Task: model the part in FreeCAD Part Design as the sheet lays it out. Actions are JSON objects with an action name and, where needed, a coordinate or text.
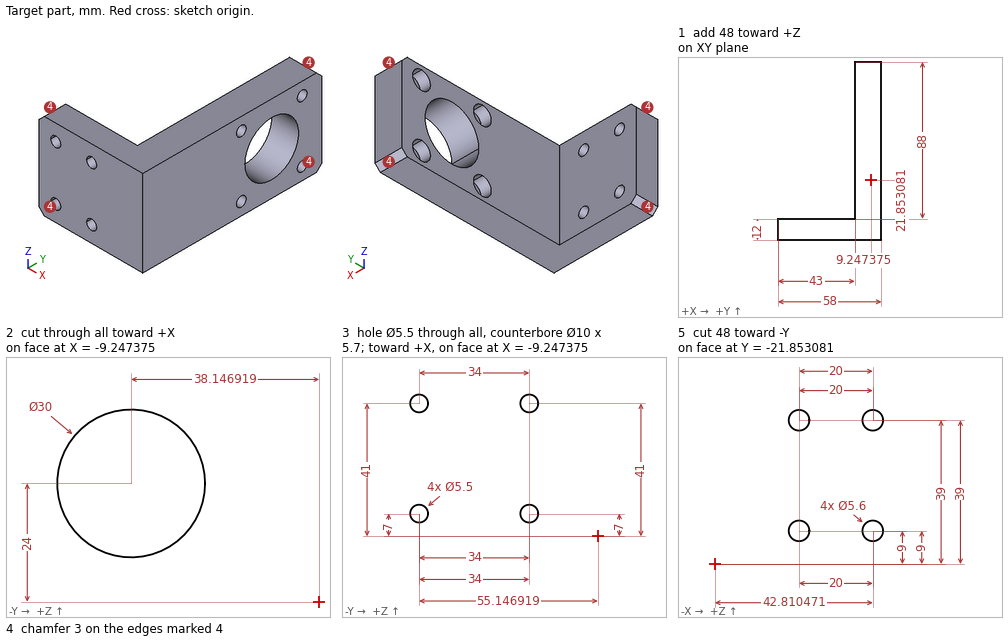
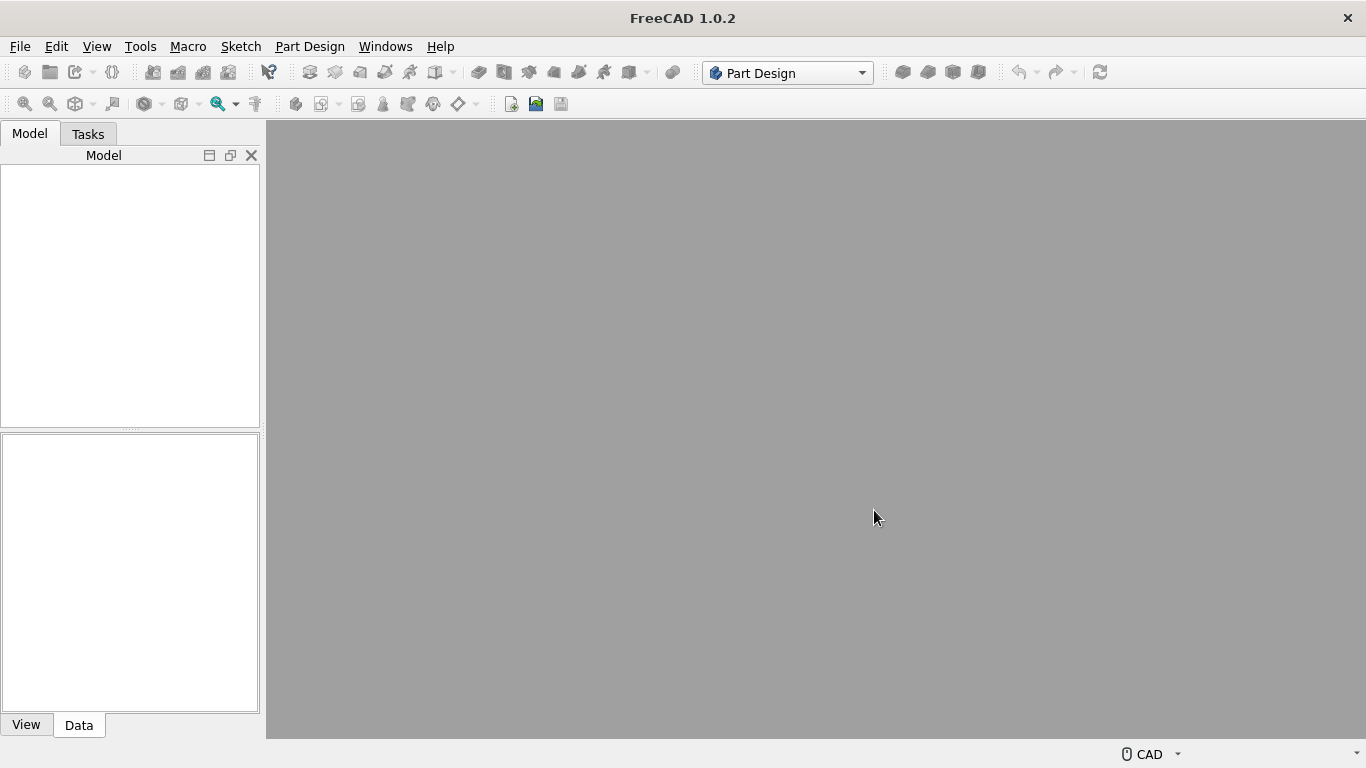
{"action": "left_click", "coordinate": [511, 104]}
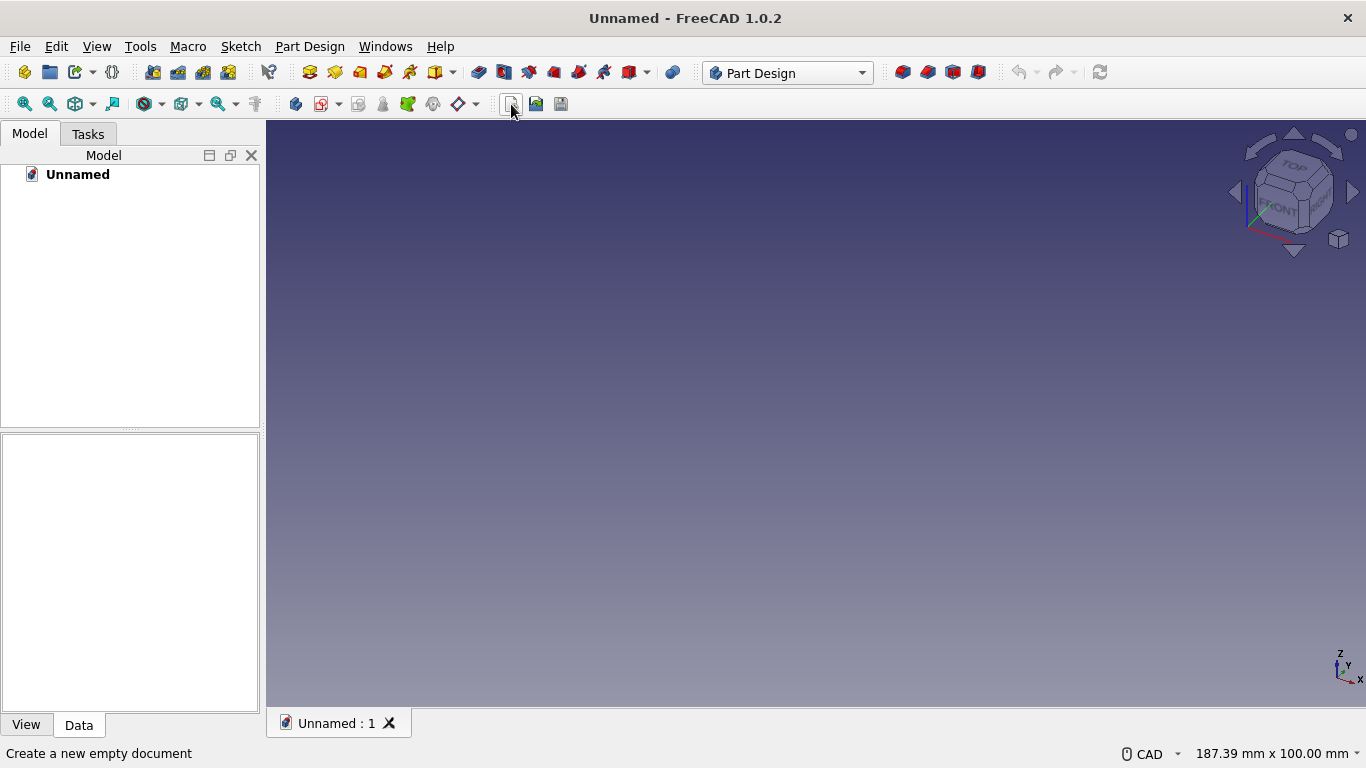
{"action": "left_click", "coordinate": [320, 104]}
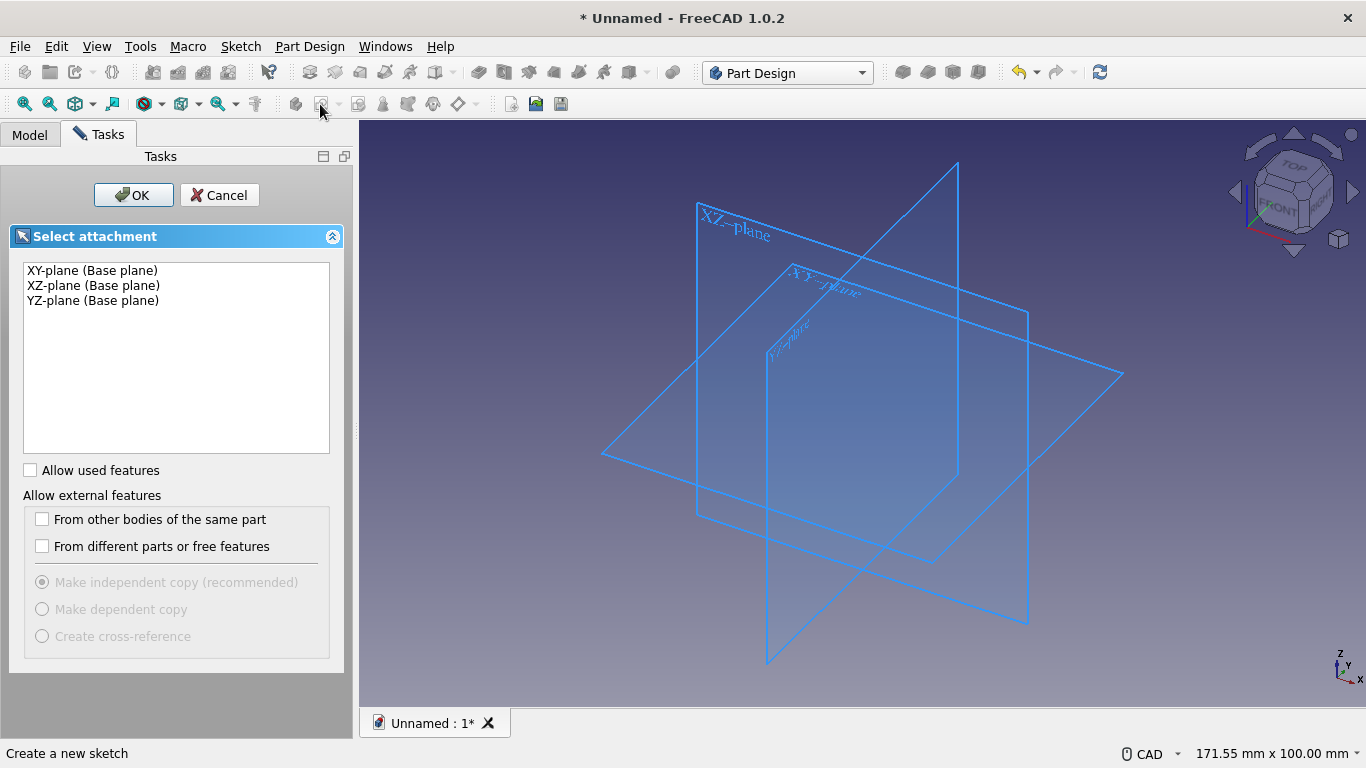
{"action": "left_click", "coordinate": [84, 270]}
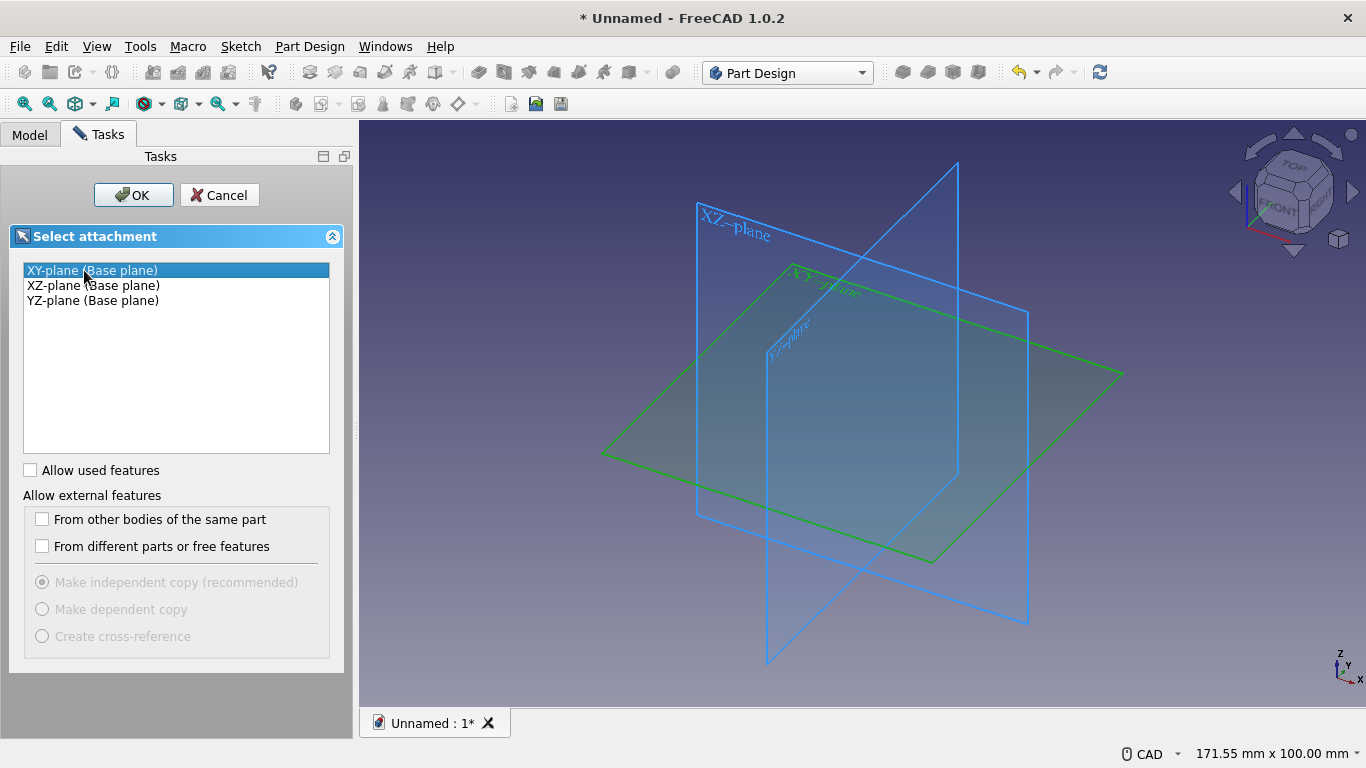
{"action": "left_click", "coordinate": [134, 195]}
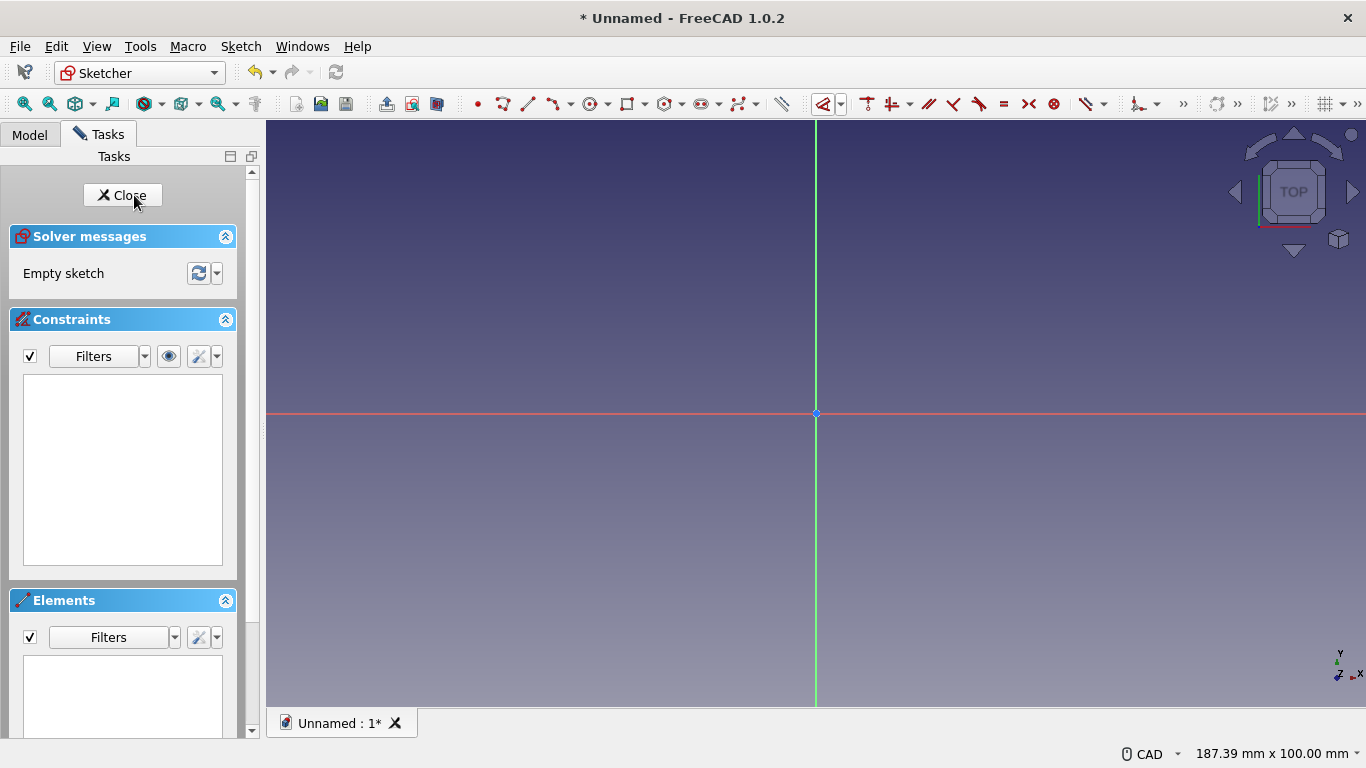
{"action": "scroll", "coordinate": [886, 606], "scroll_direction": "down", "scroll_amount": 2}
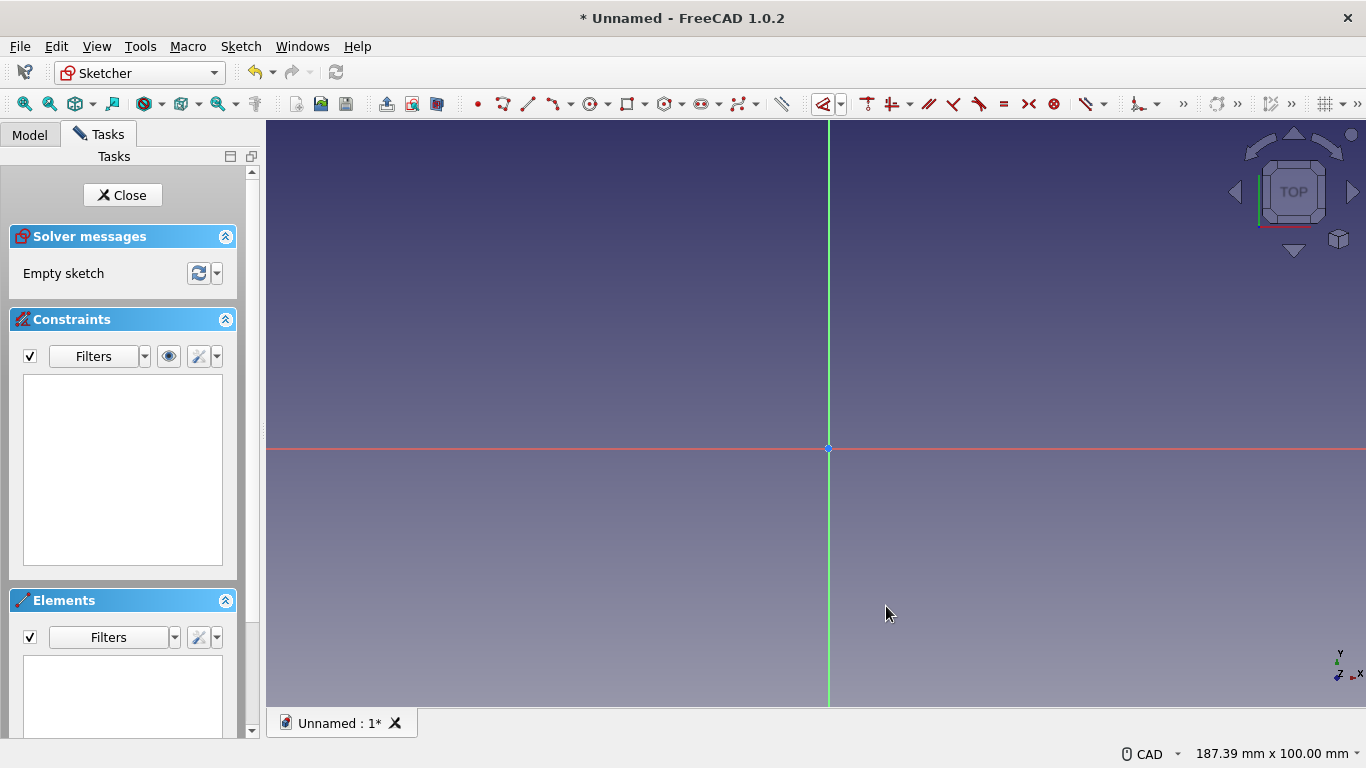
{"action": "left_click", "coordinate": [503, 104]}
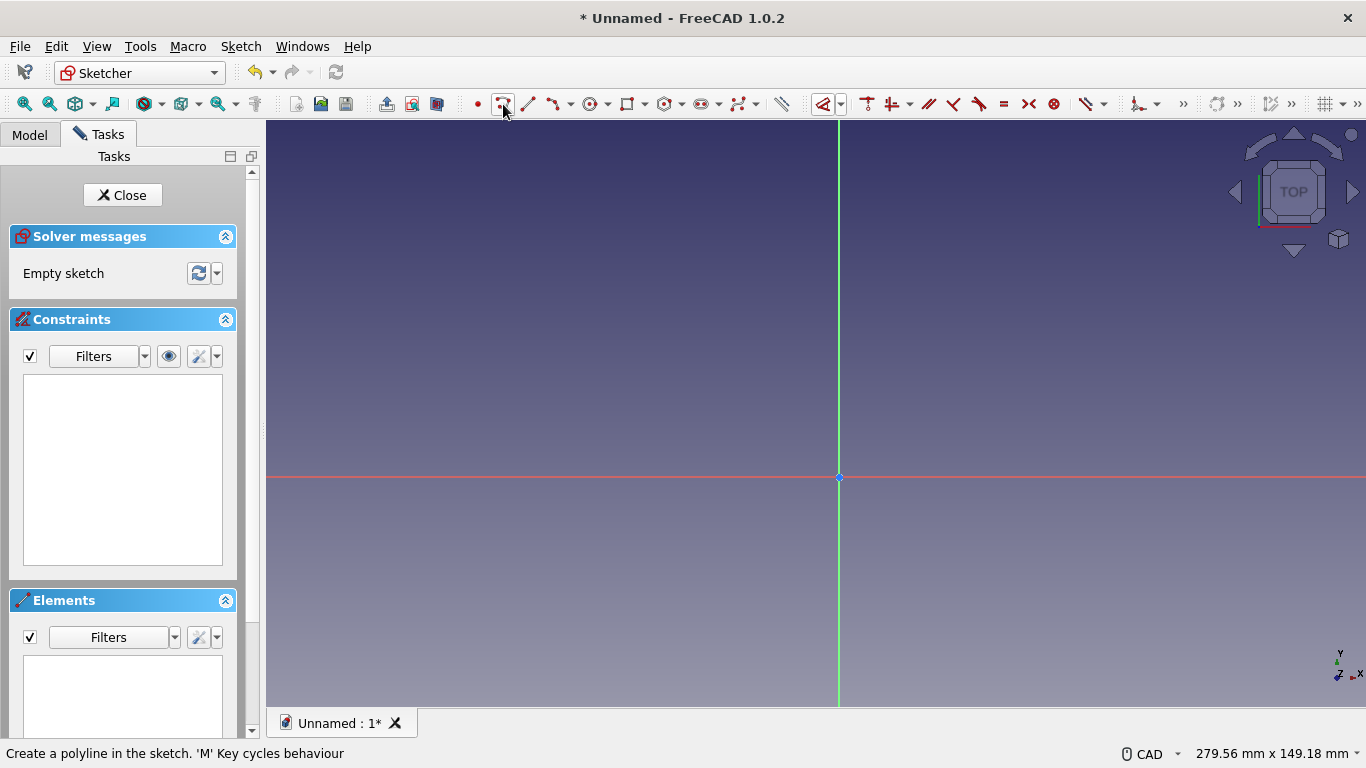
{"action": "left_click", "coordinate": [803, 563]}
{"action": "left_click", "coordinate": [634, 563]}
{"action": "left_click", "coordinate": [634, 610]}
{"action": "left_click", "coordinate": [862, 610]}
{"action": "left_click", "coordinate": [862, 217]}
{"action": "left_click", "coordinate": [803, 217]}
{"action": "left_click", "coordinate": [803, 564]}
{"action": "key", "text": "Escape"}
{"action": "key", "text": "Escape"}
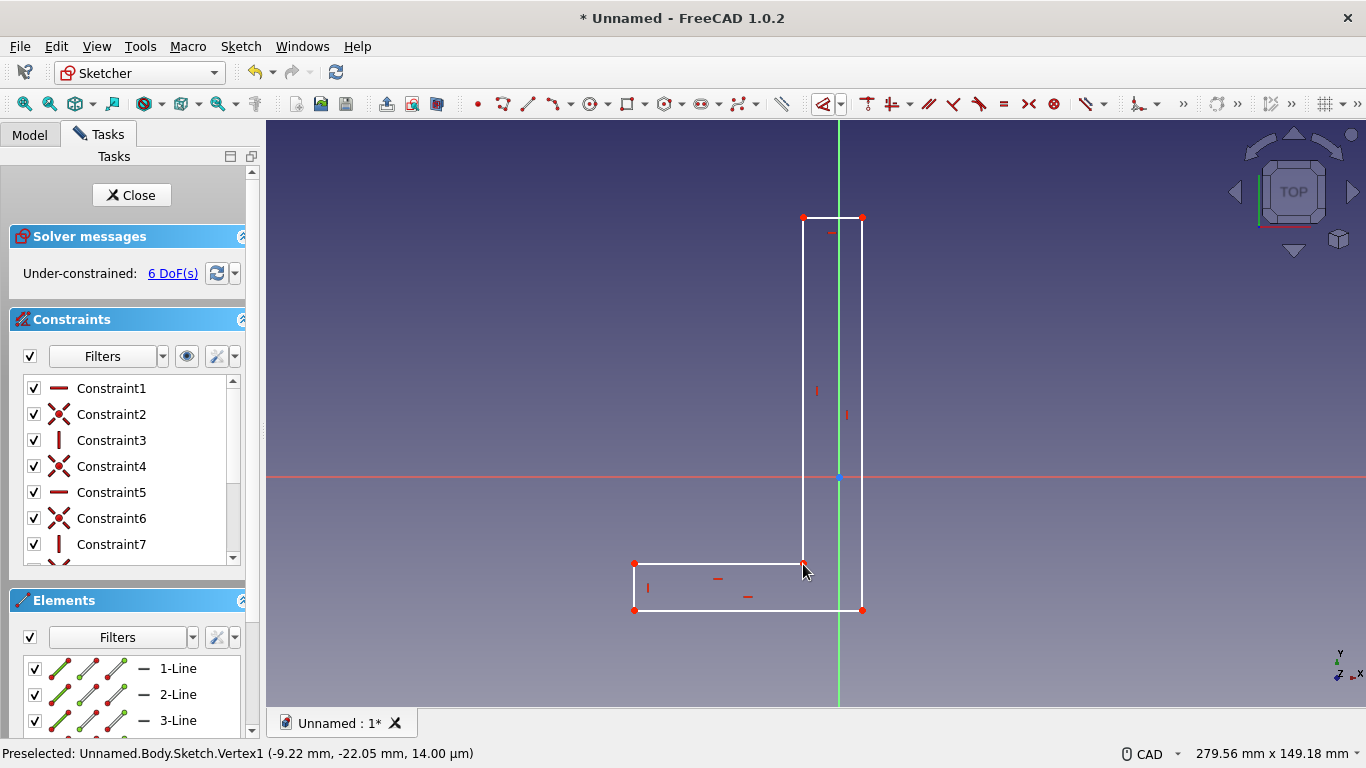
{"action": "left_click", "coordinate": [822, 104]}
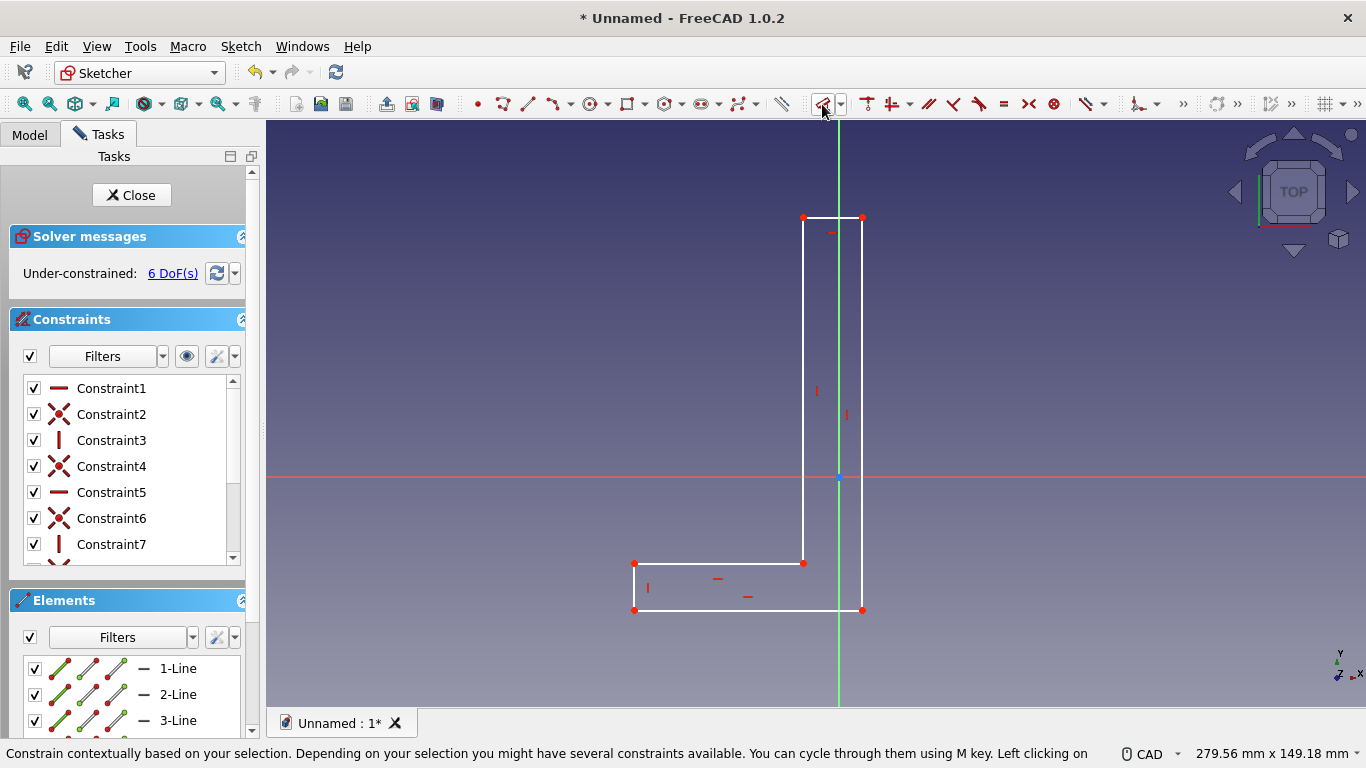
{"action": "left_click", "coordinate": [752, 564]}
{"action": "left_click", "coordinate": [719, 530]}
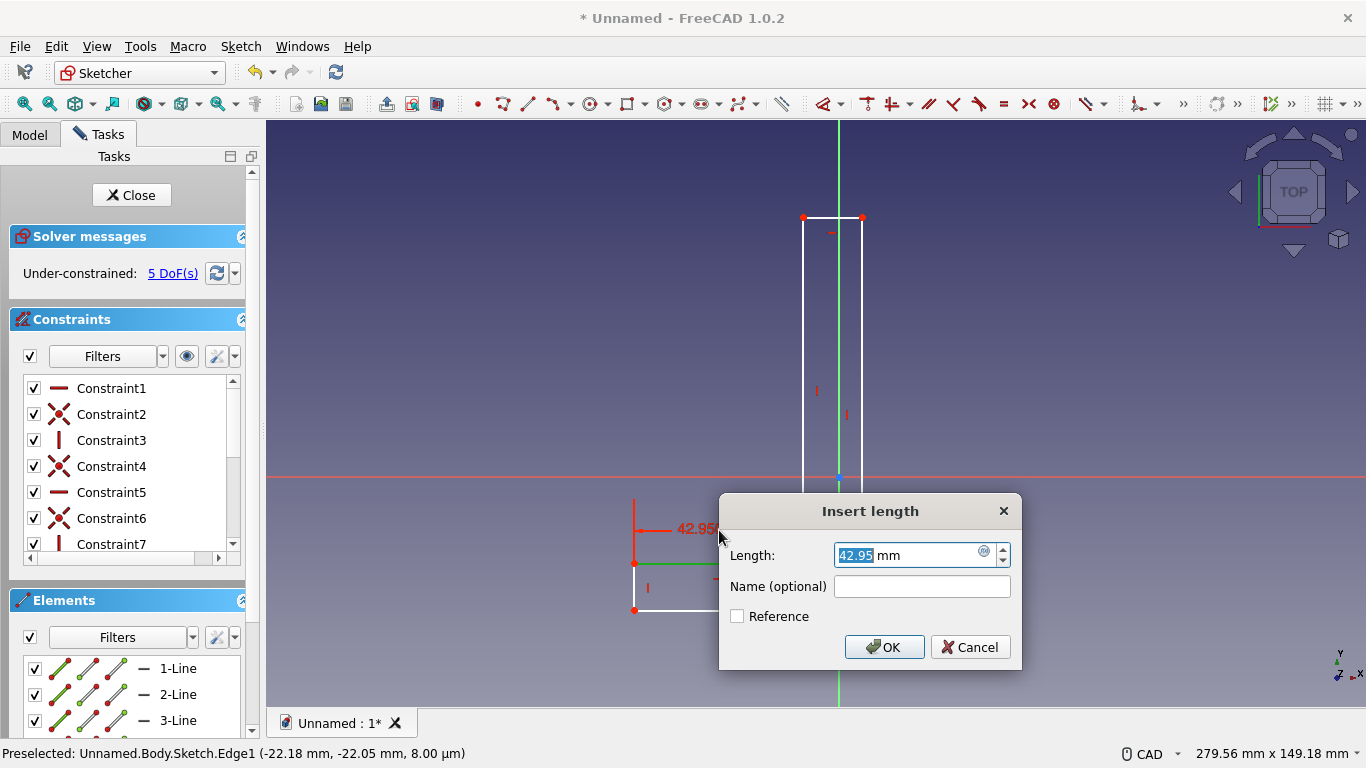
{"action": "type", "text": "43"}
{"action": "key", "text": "Return"}